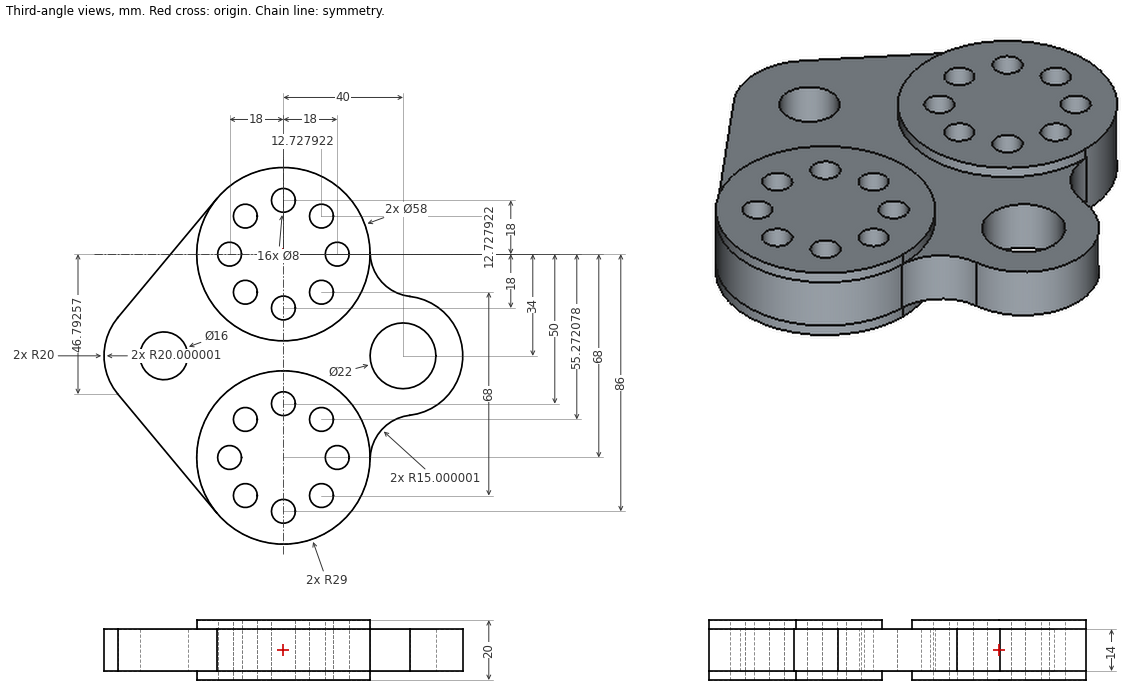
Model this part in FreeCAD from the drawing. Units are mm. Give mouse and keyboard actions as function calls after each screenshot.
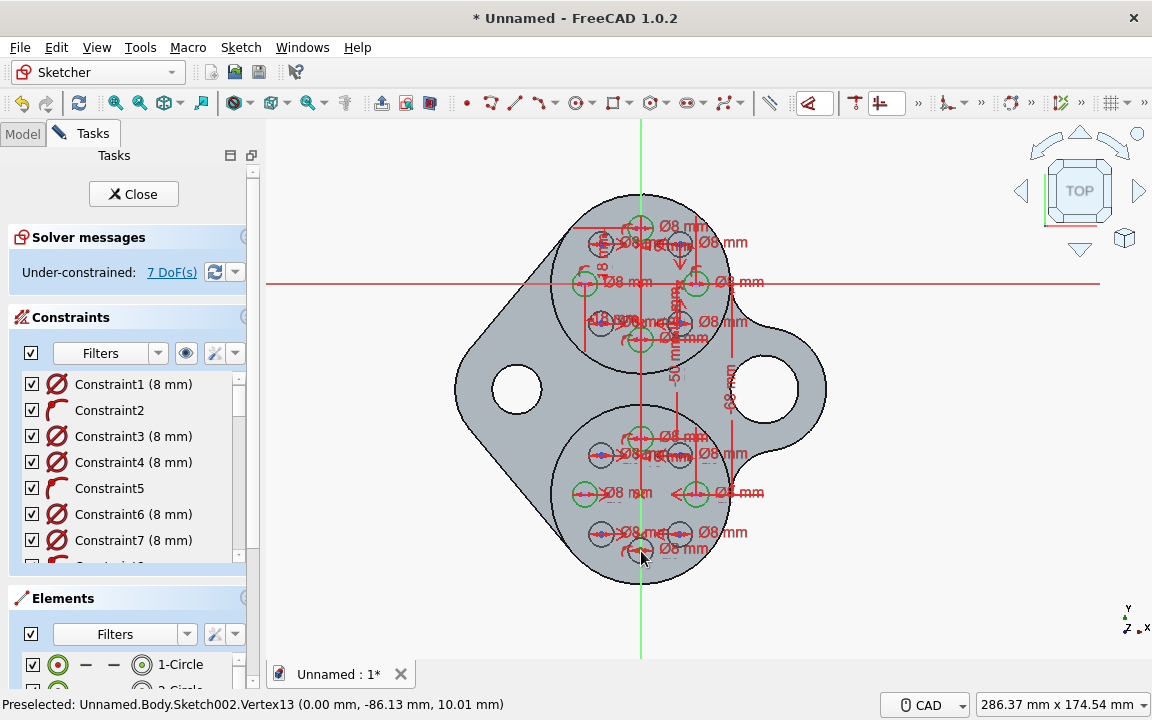
key(i)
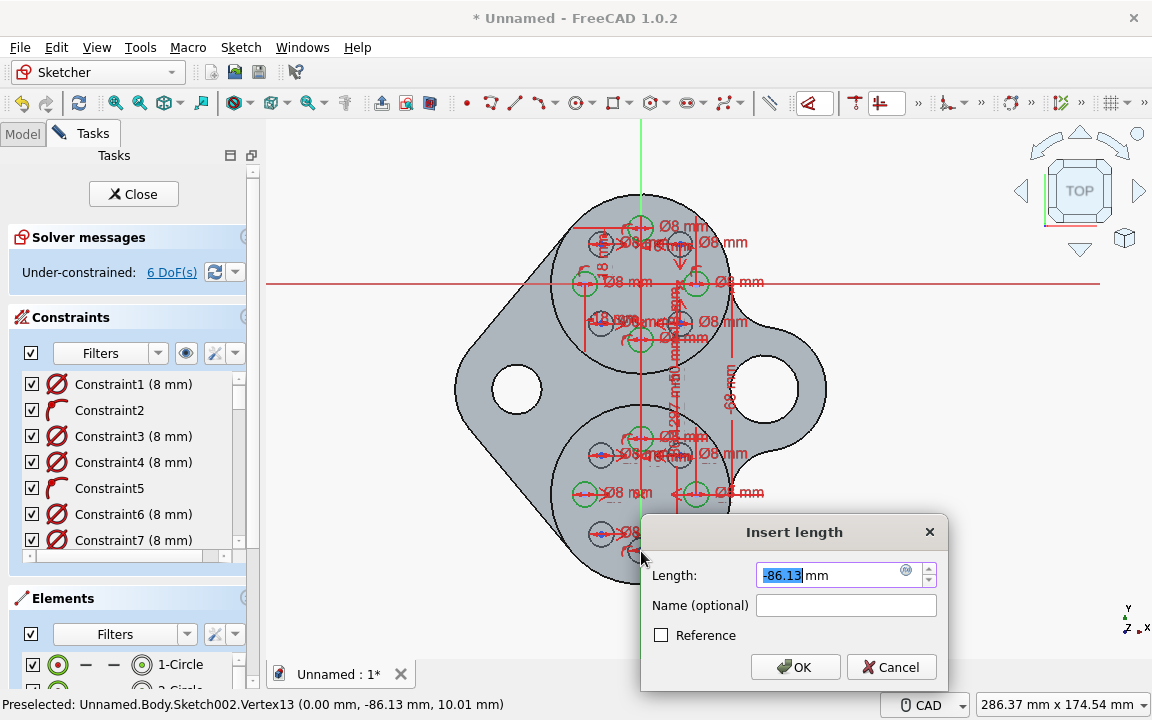
text(-86)
key(Return)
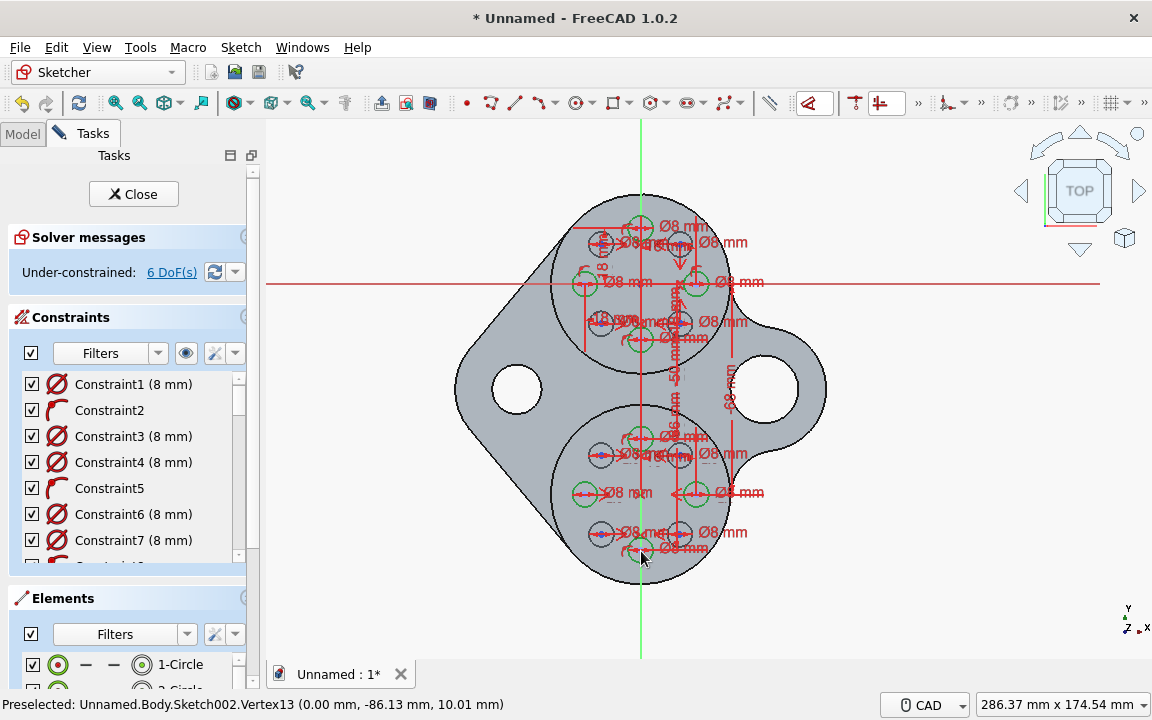
click(680, 324)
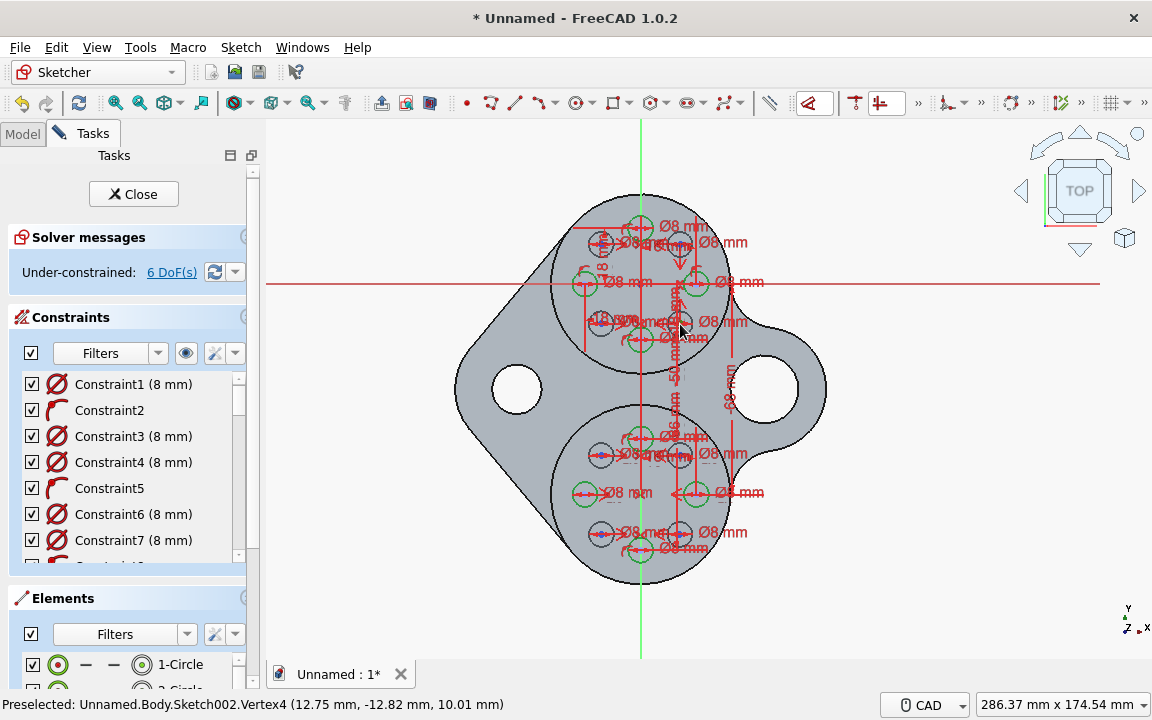
click(680, 534)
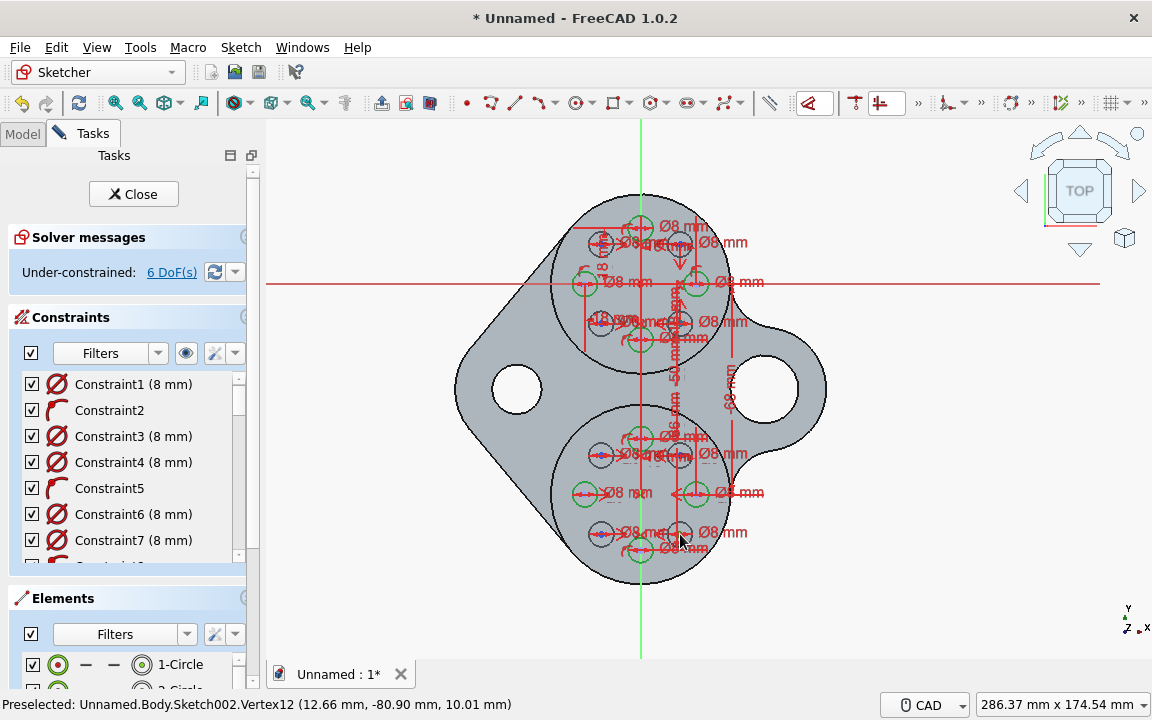
key(i)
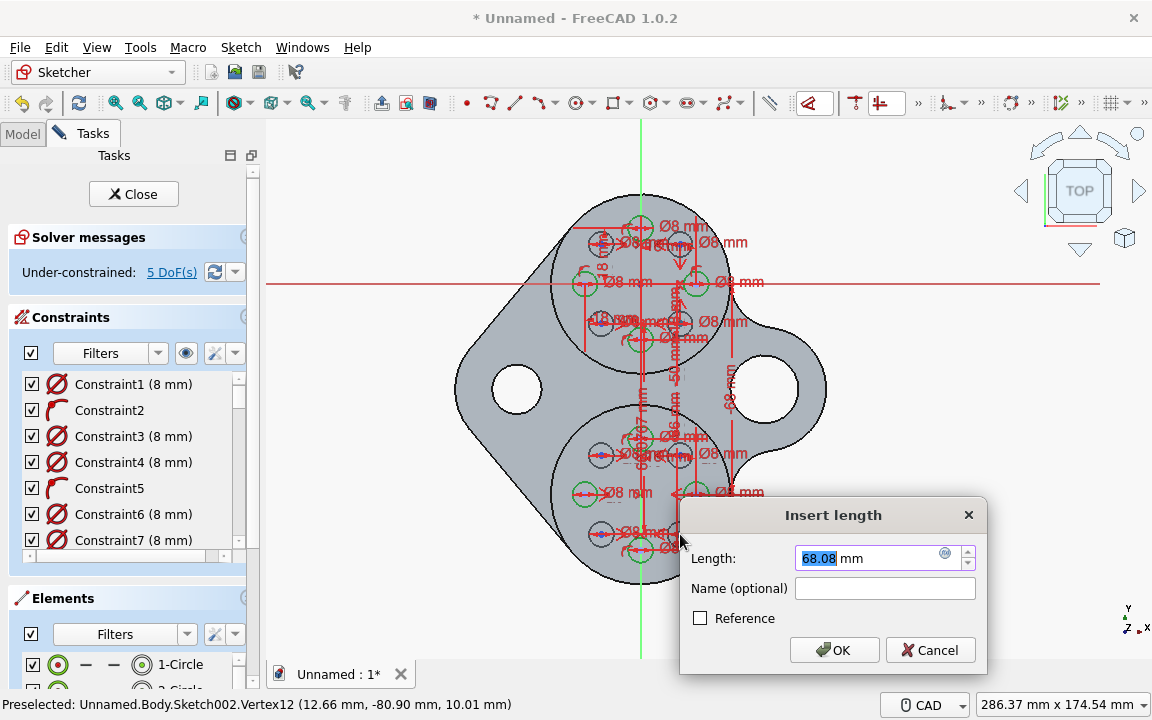
text(68)
key(Return)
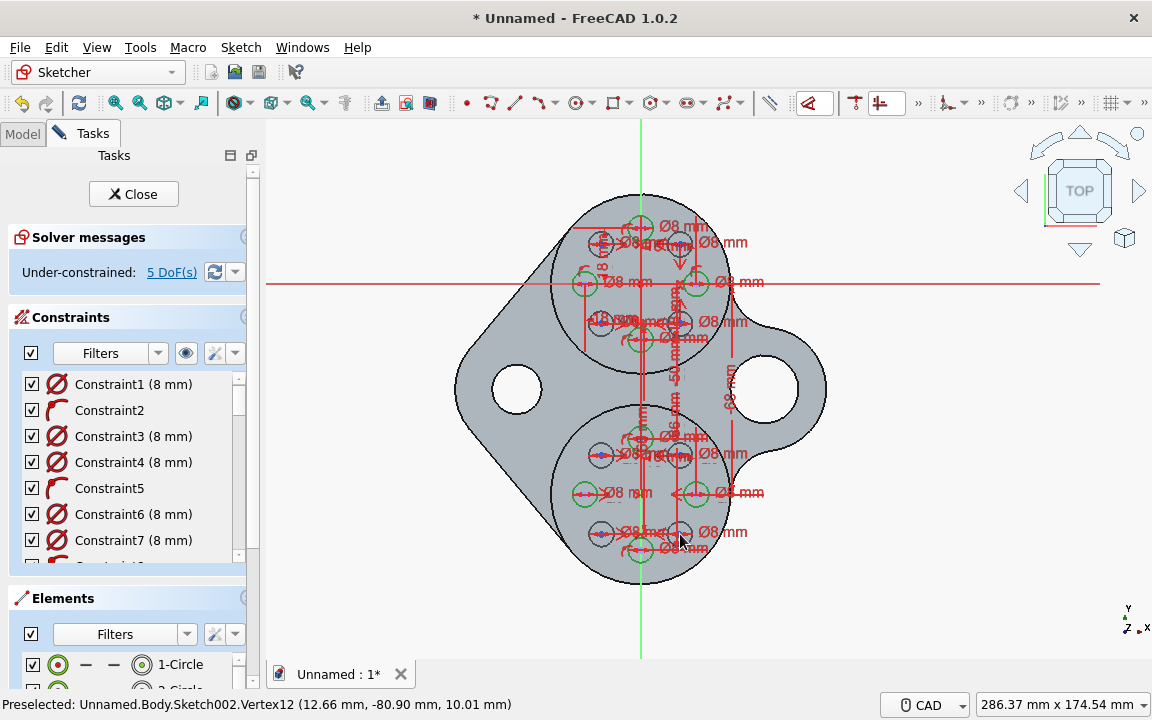
click(680, 244)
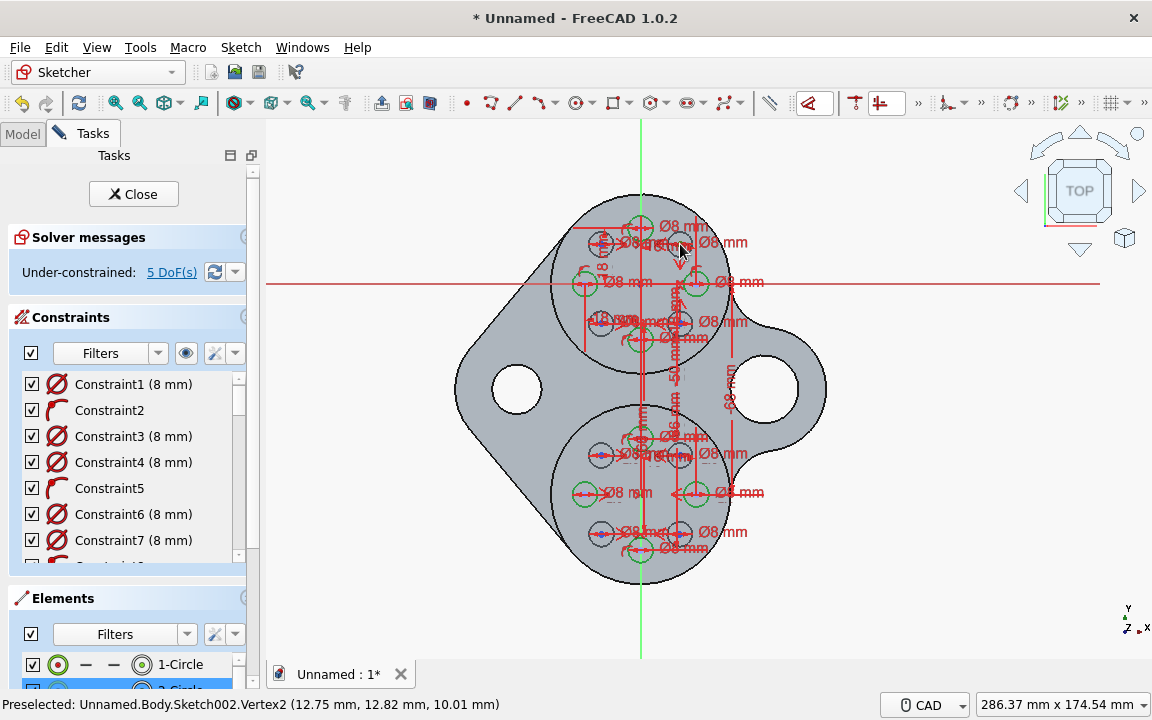
key(l)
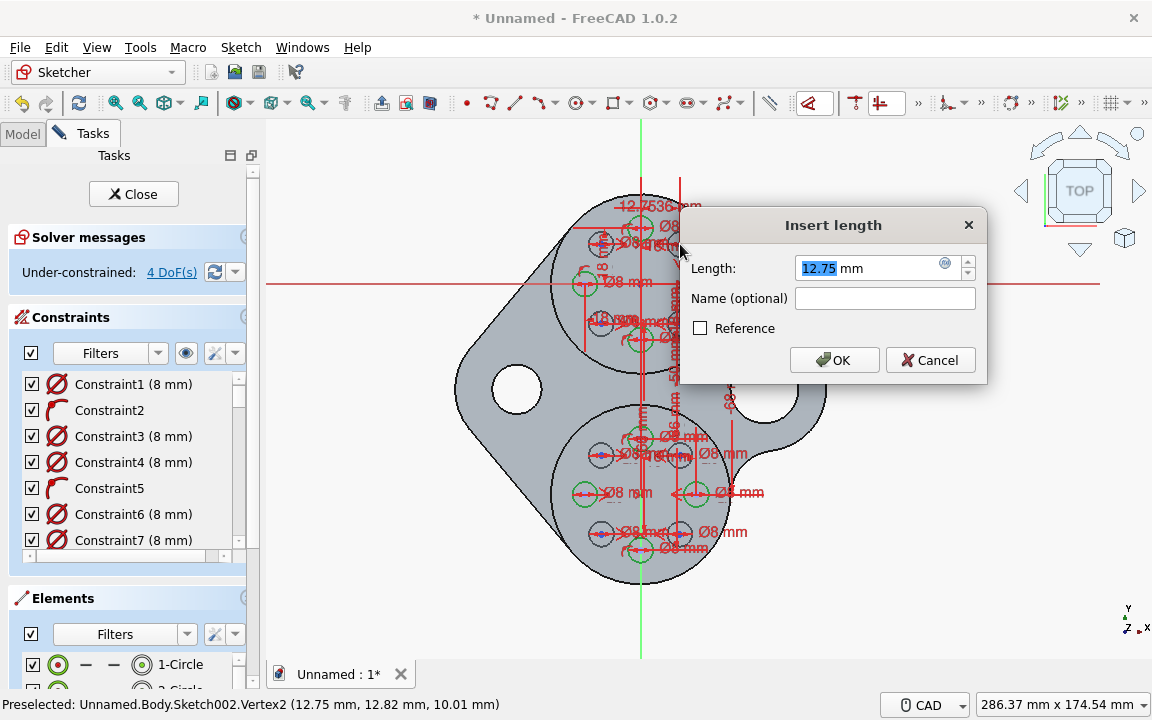
text(12.727922)
key(Return)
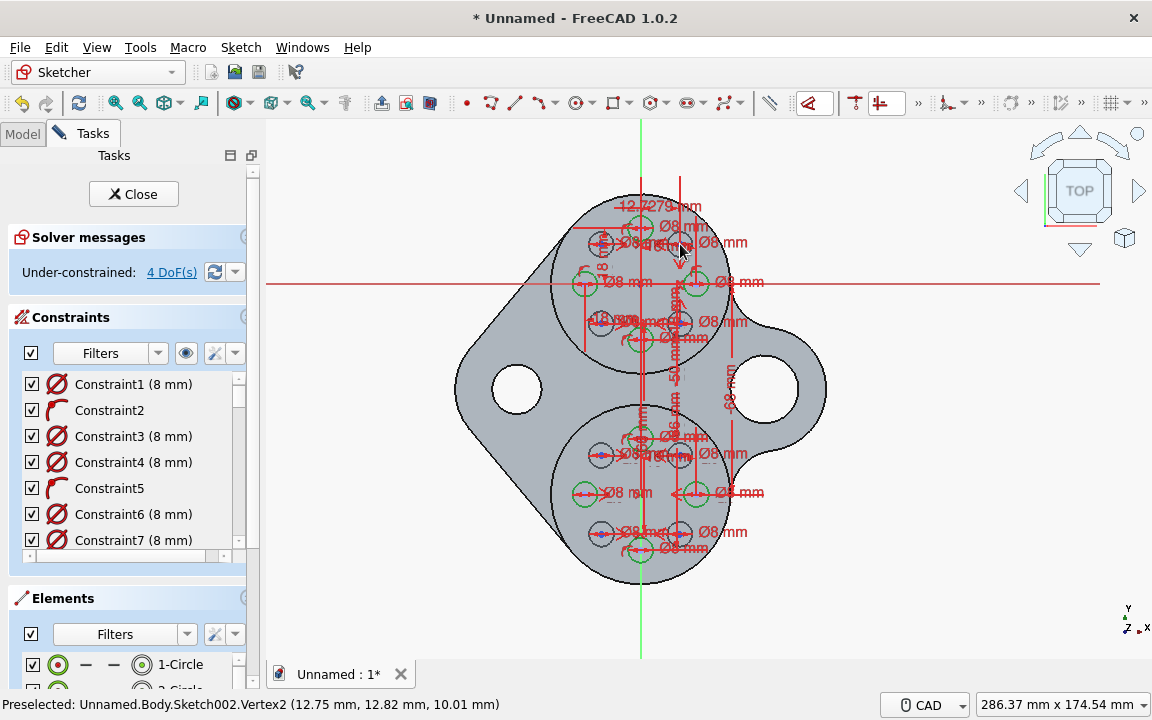
click(680, 244)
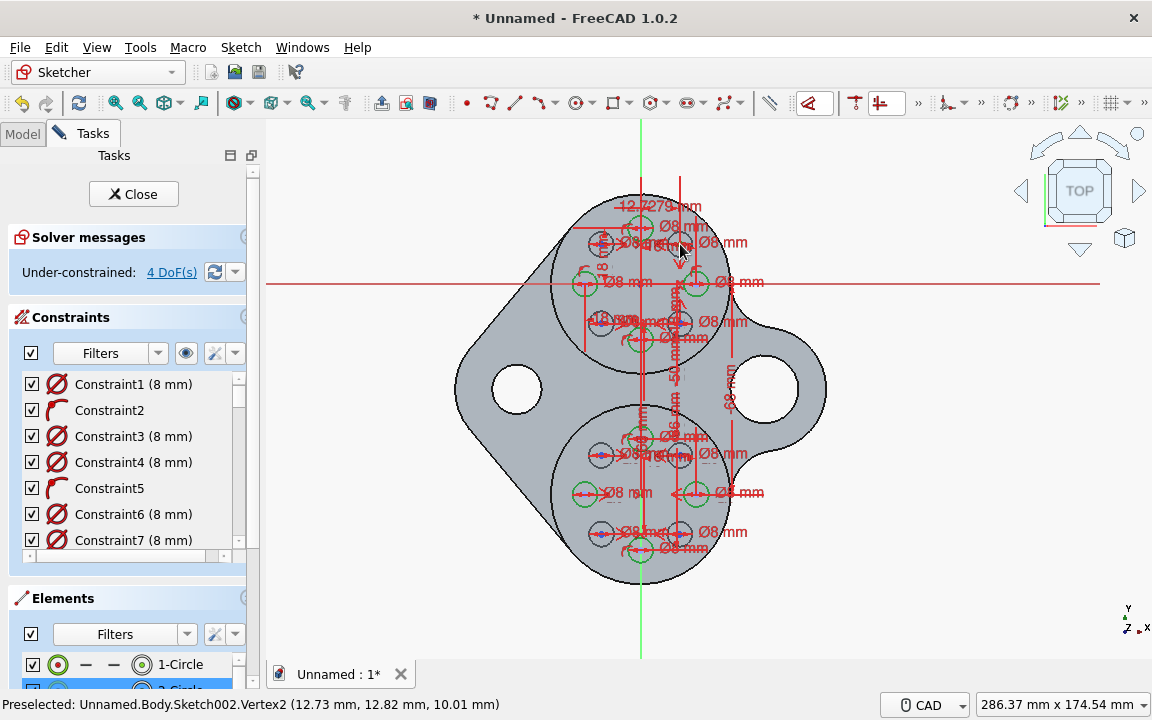
key(i)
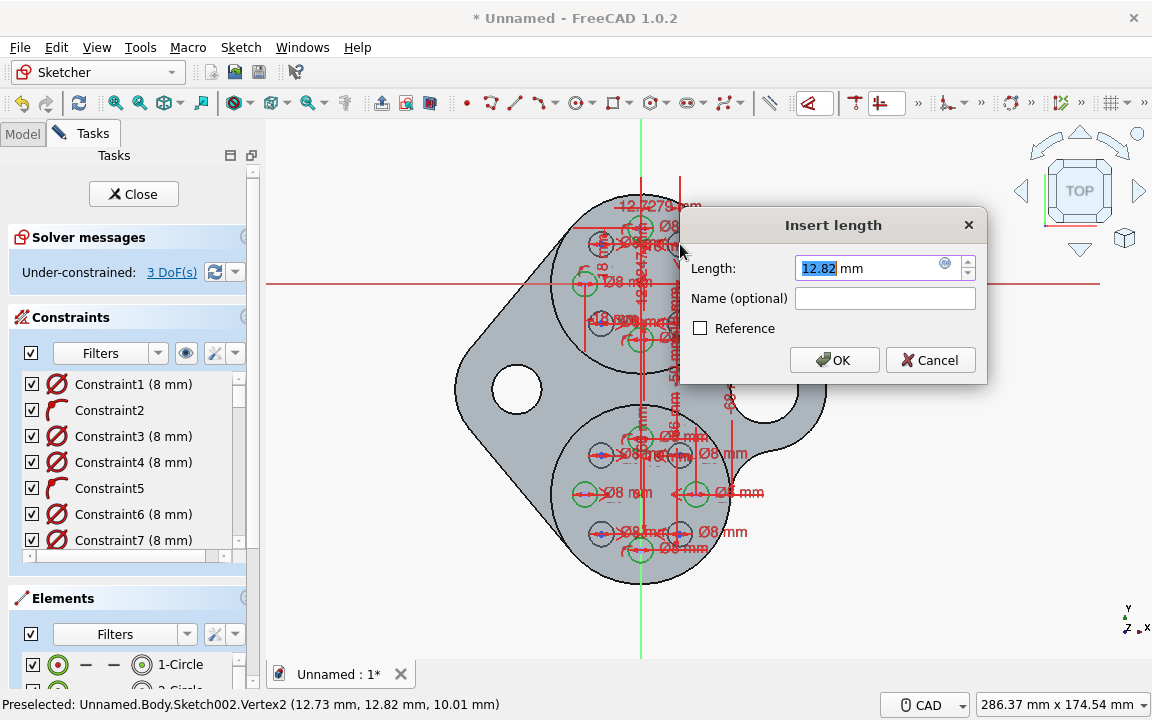
text(12.727922)
key(Return)